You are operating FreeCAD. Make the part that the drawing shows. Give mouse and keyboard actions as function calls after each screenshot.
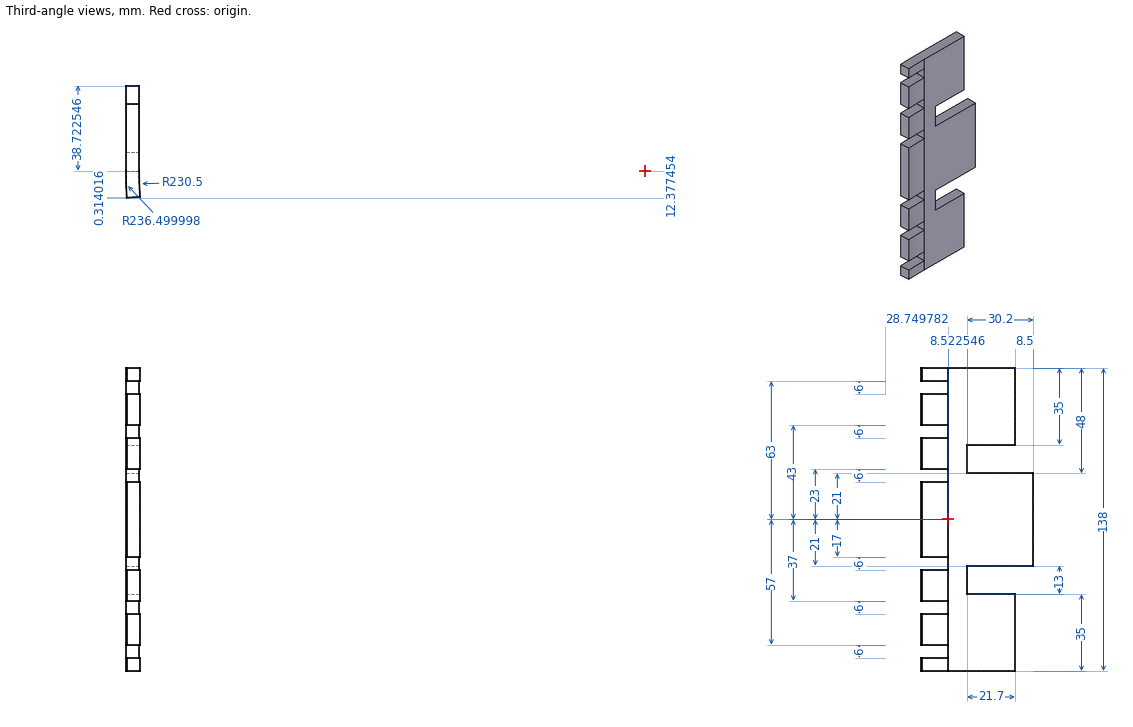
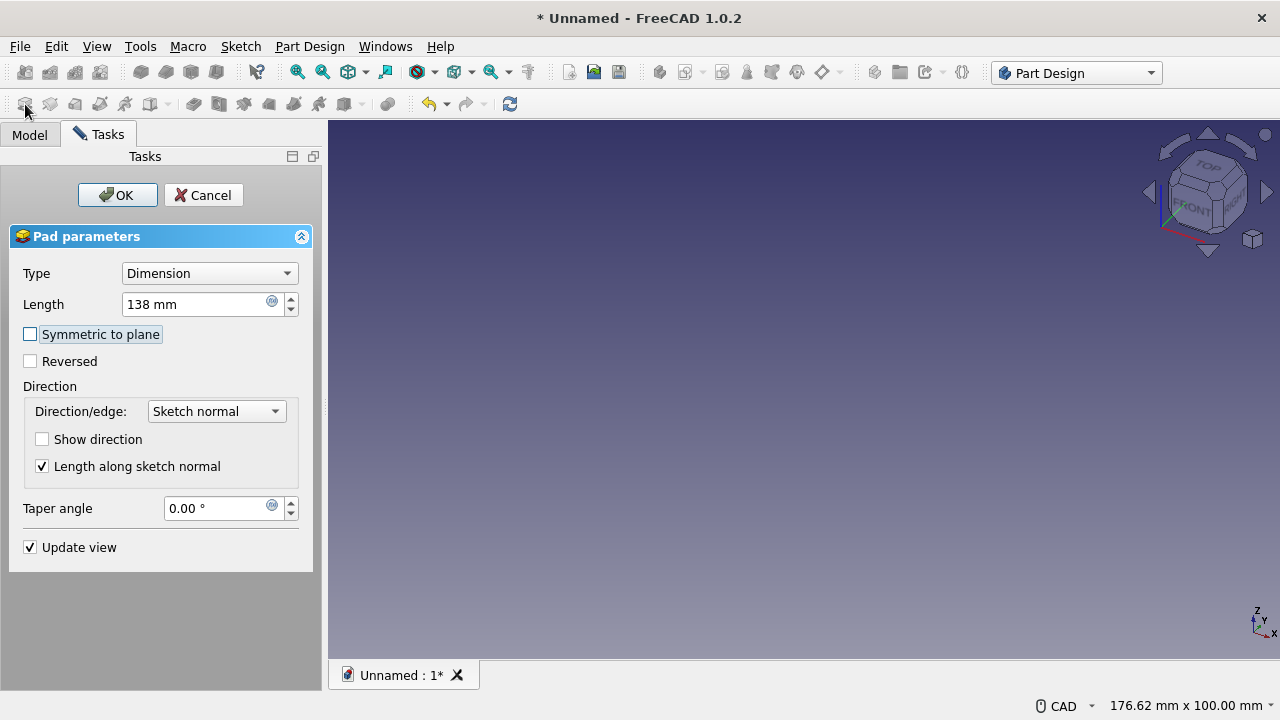
click(31, 334)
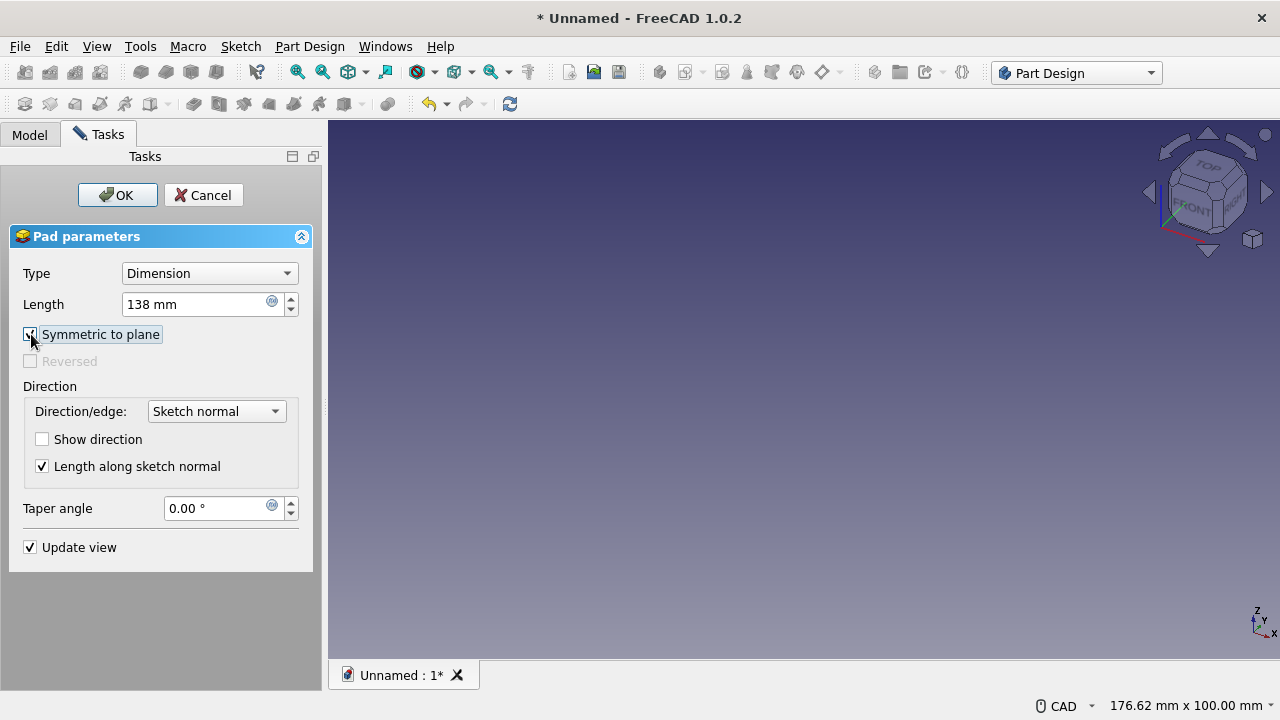
click(118, 195)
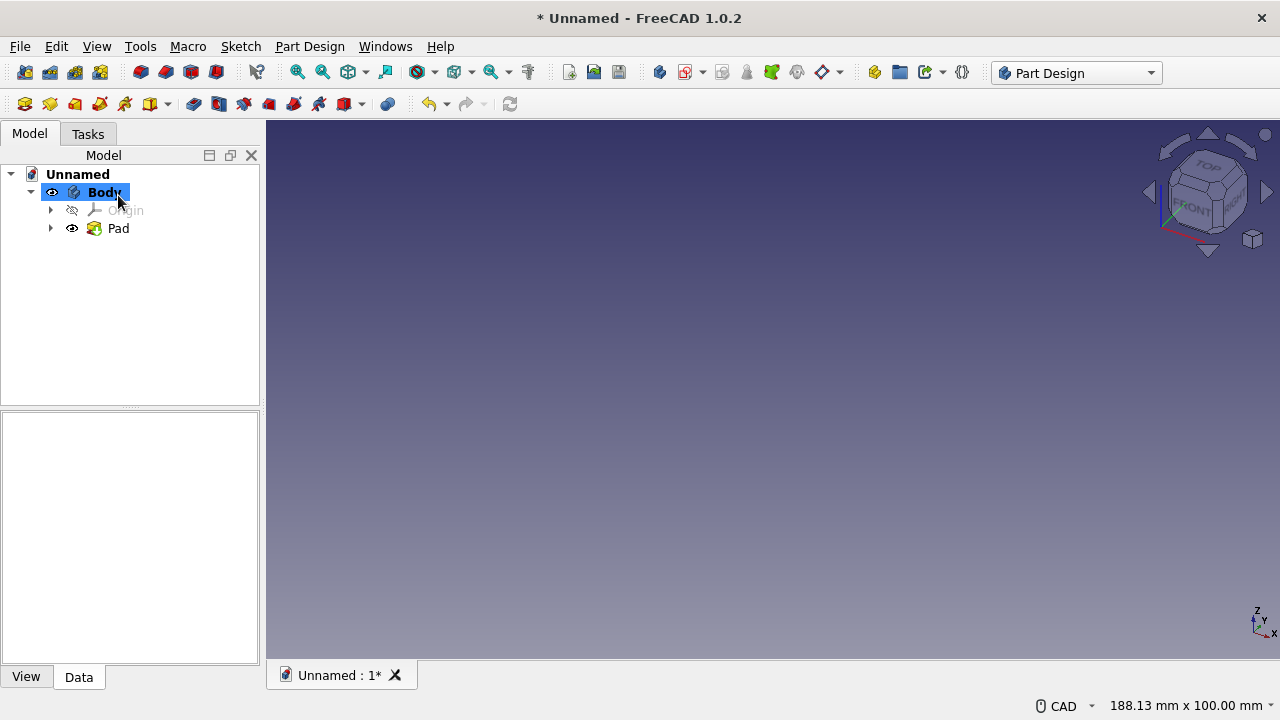
key(v)
key(f)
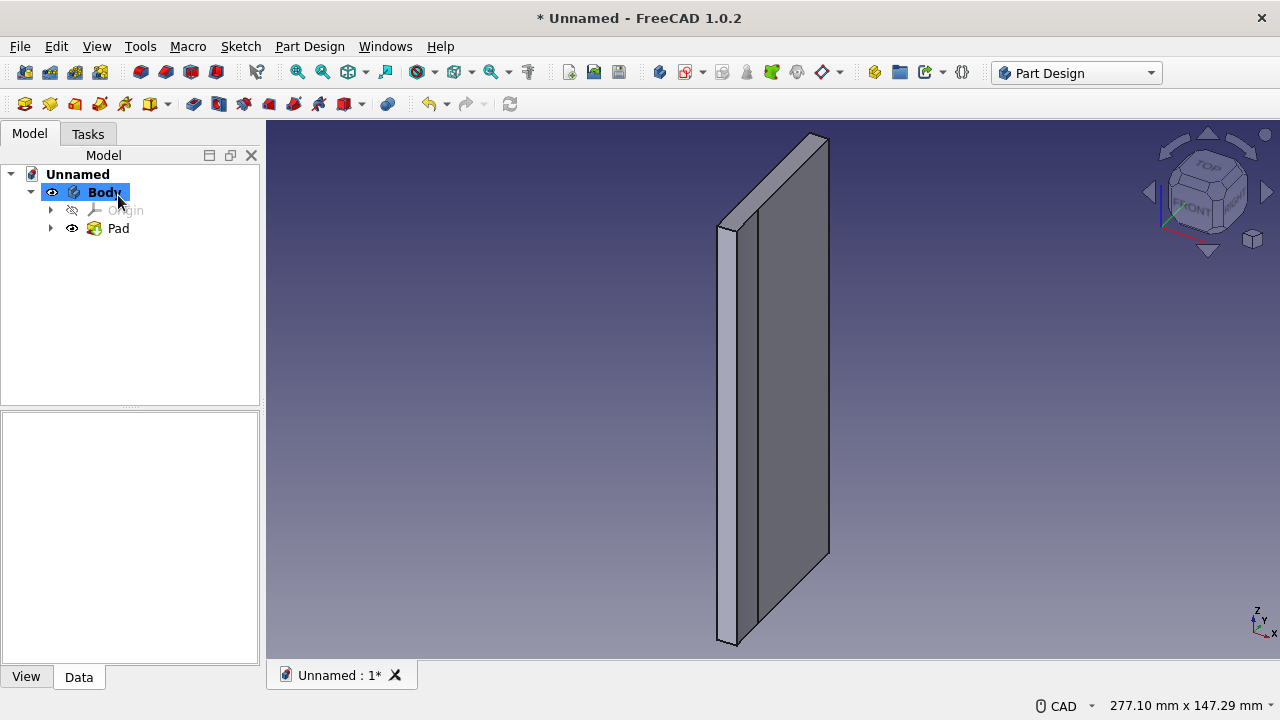
click(684, 72)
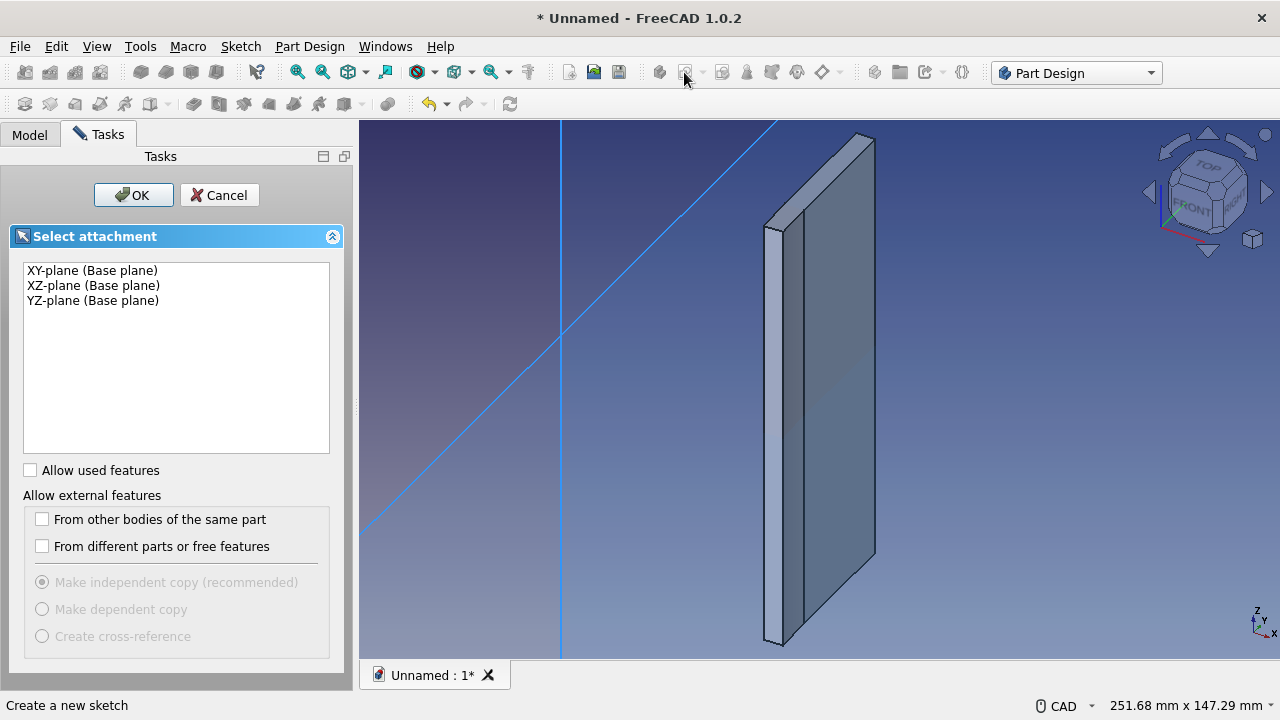
click(84, 300)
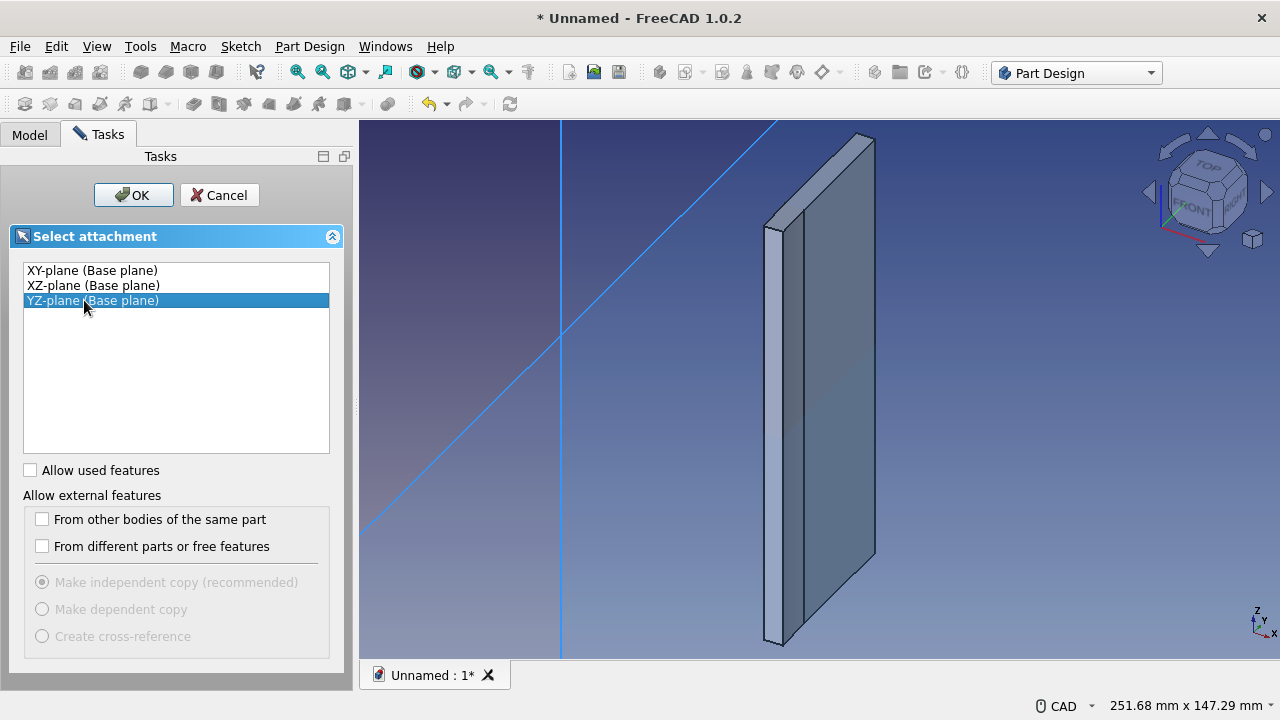
click(134, 195)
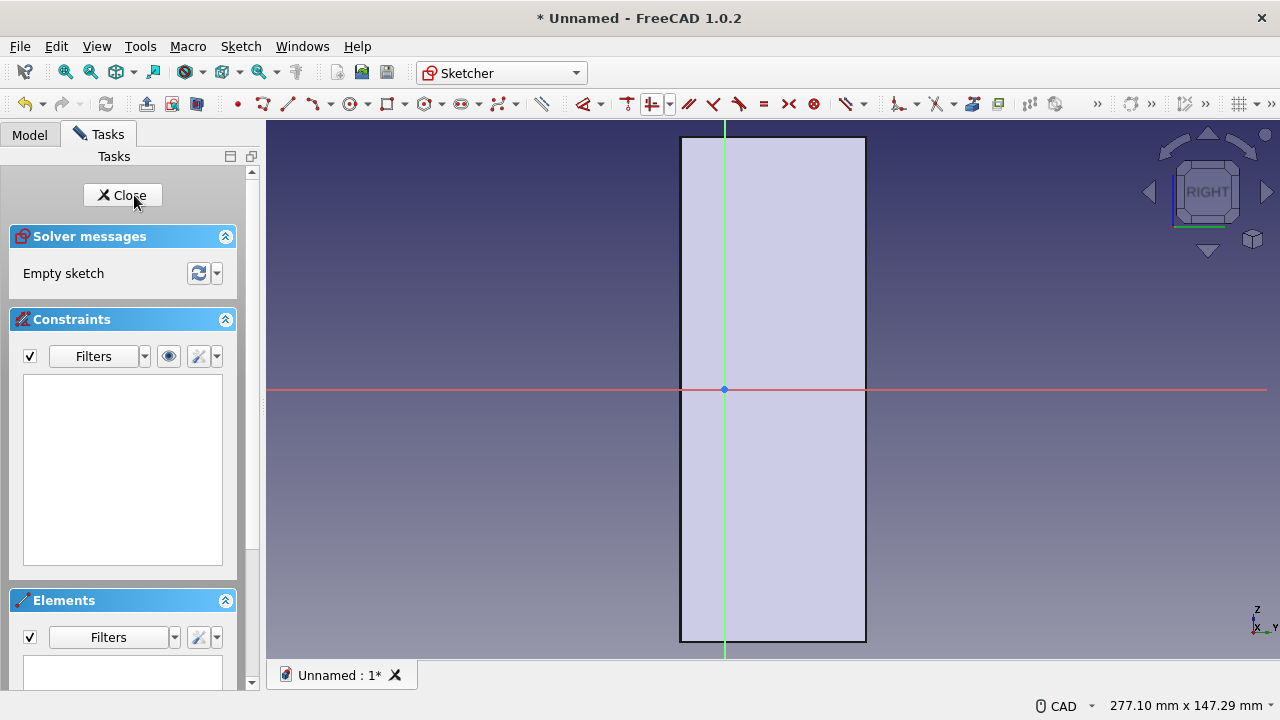
scroll(770, 390, down, 2)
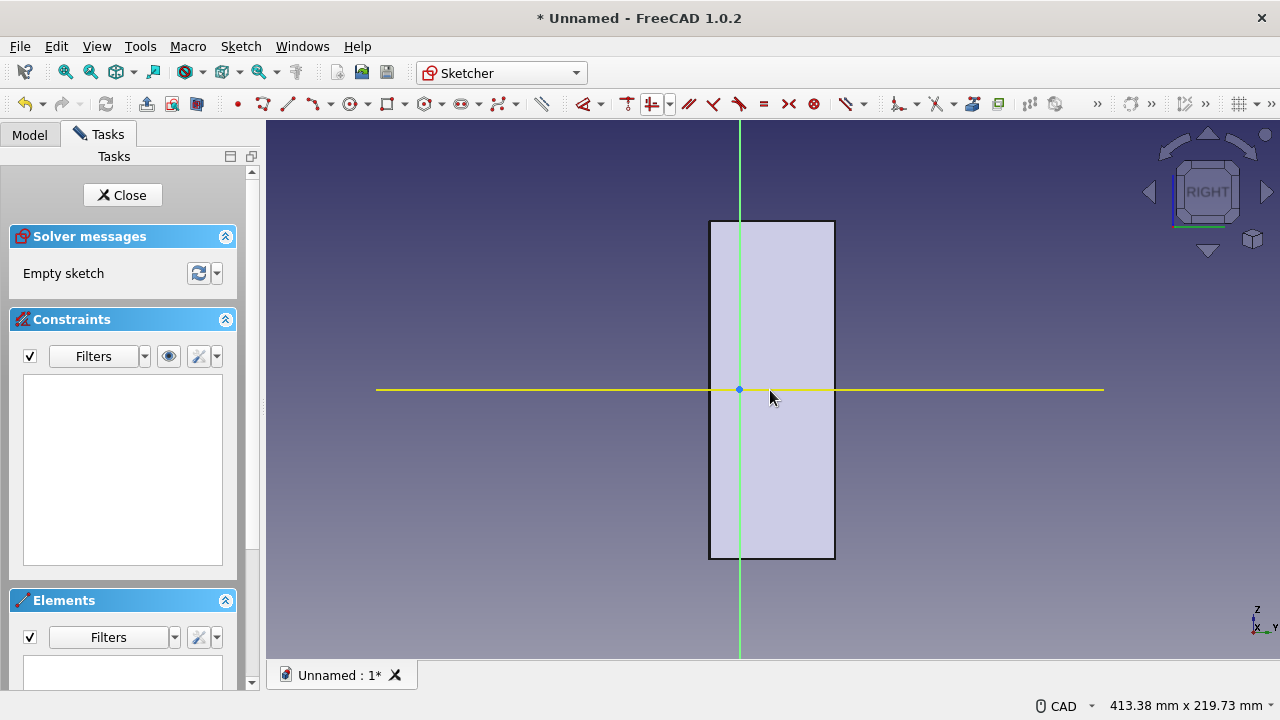
key(g)
key(r)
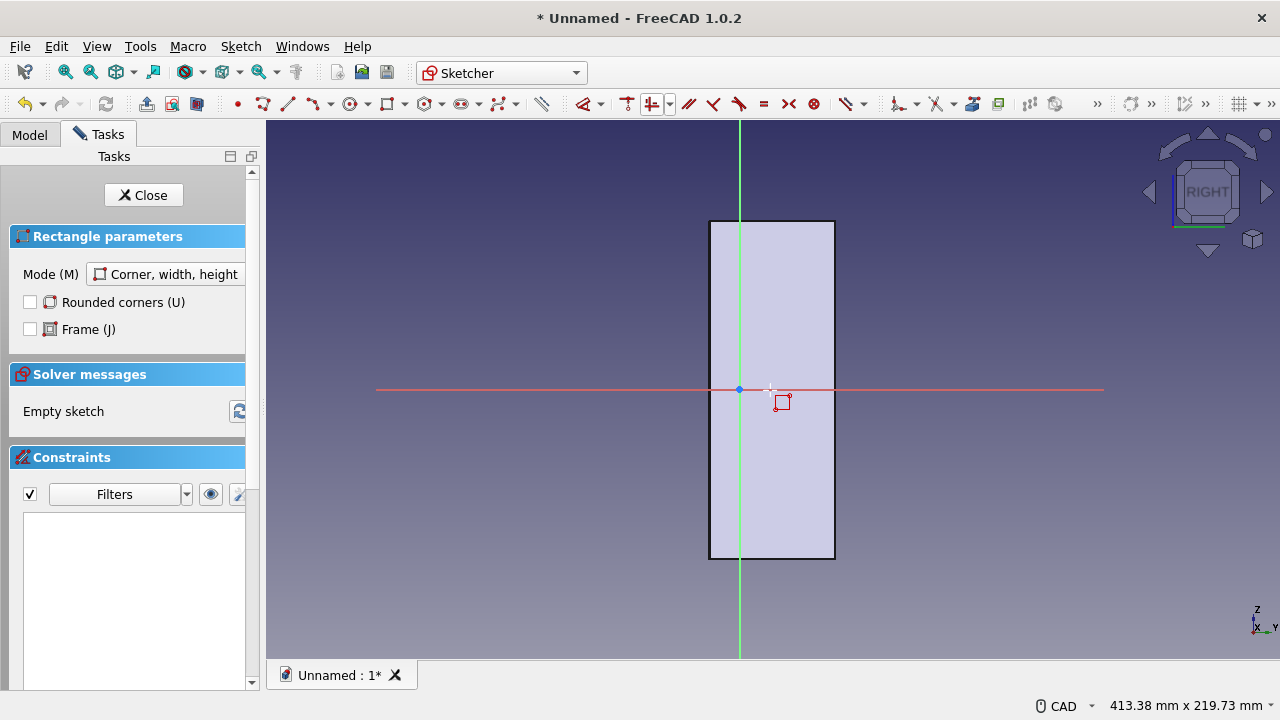
click(669, 235)
click(740, 250)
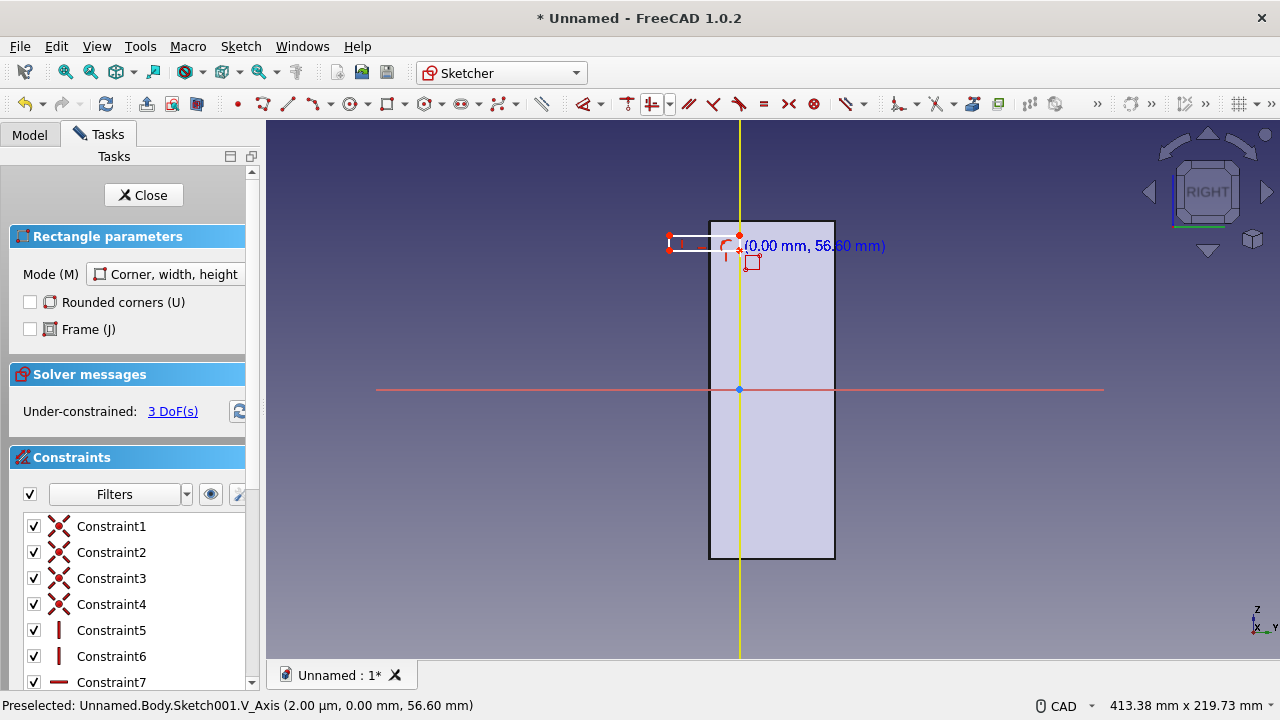
click(669, 284)
click(740, 299)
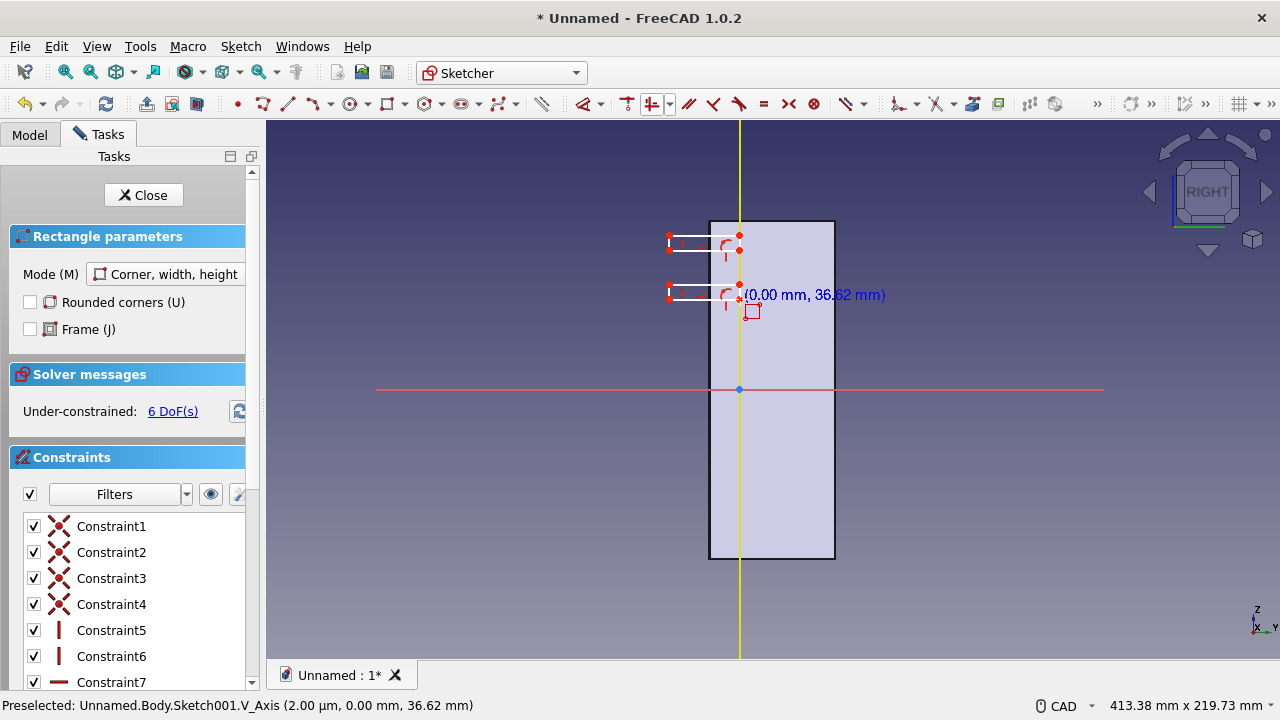
click(669, 333)
click(740, 348)